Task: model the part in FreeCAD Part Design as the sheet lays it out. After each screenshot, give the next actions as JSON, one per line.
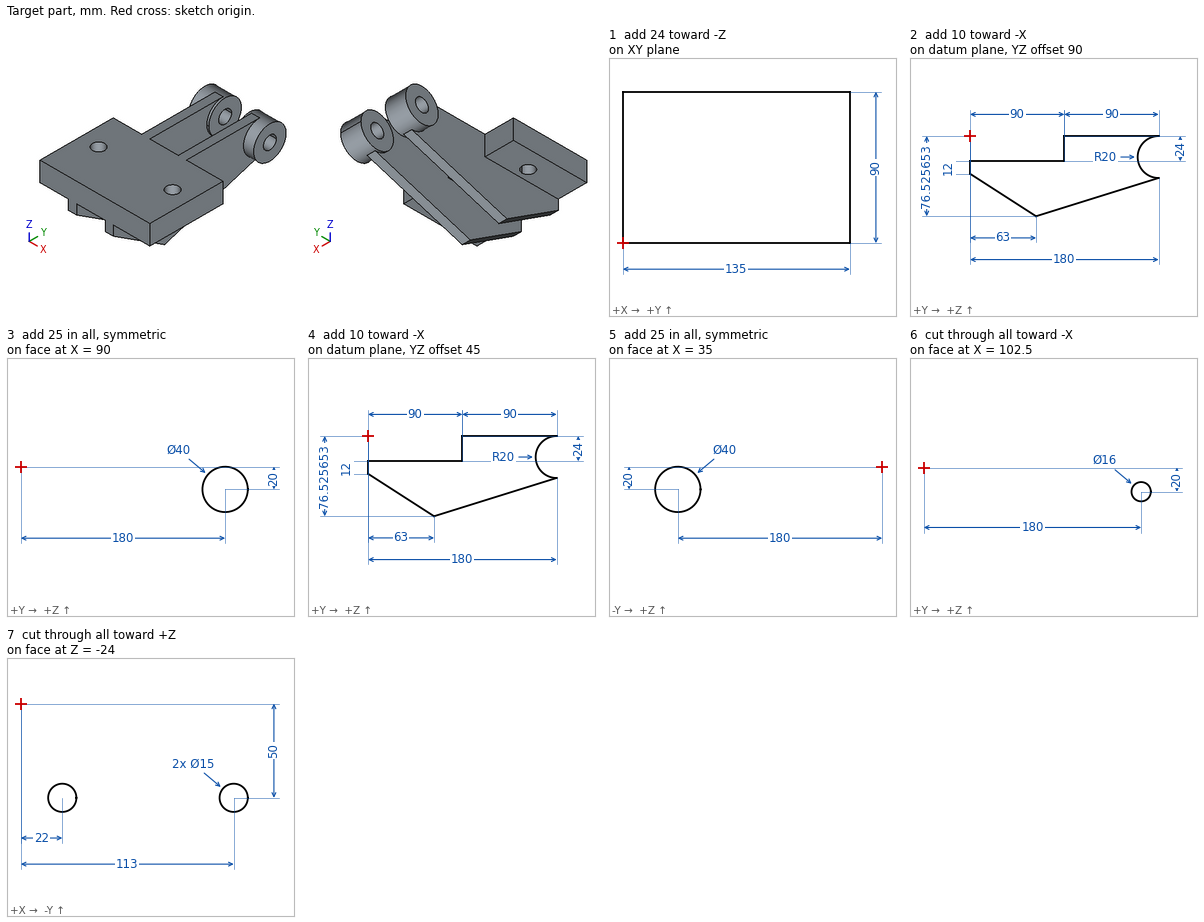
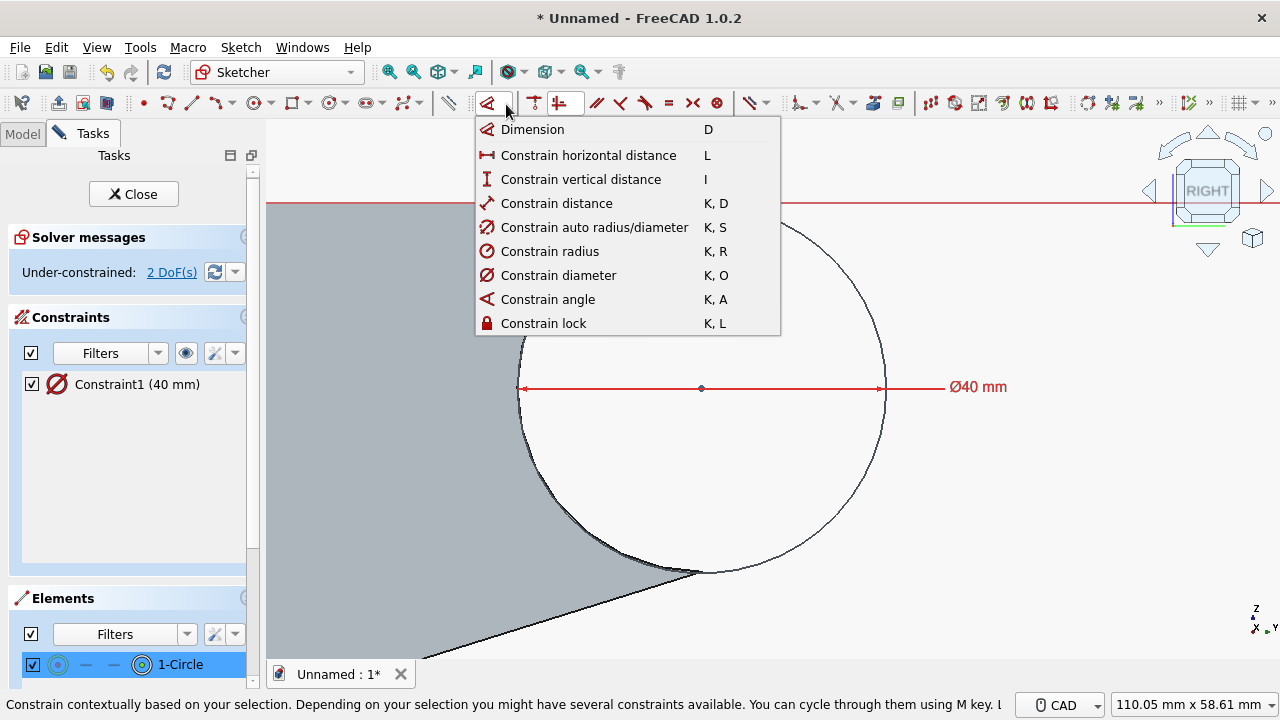
{"action": "left_click", "coordinate": [628, 179]}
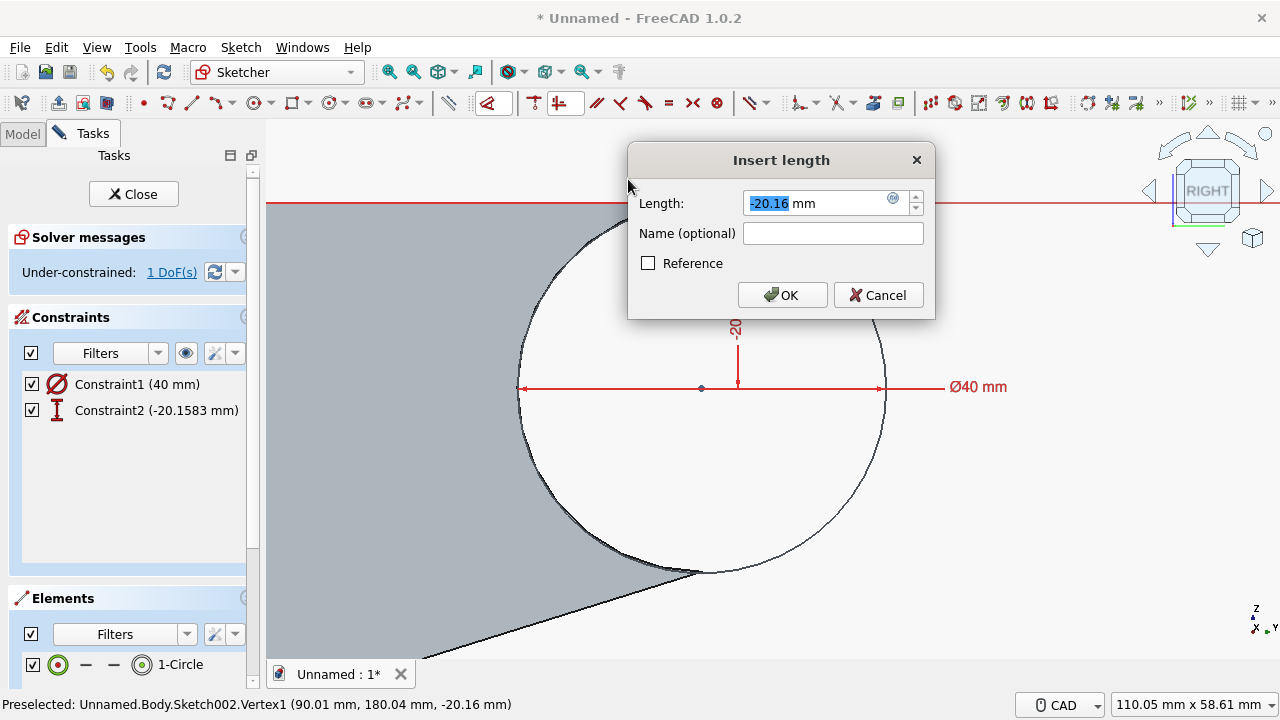
{"action": "type", "text": "-20"}
{"action": "key", "text": "Return"}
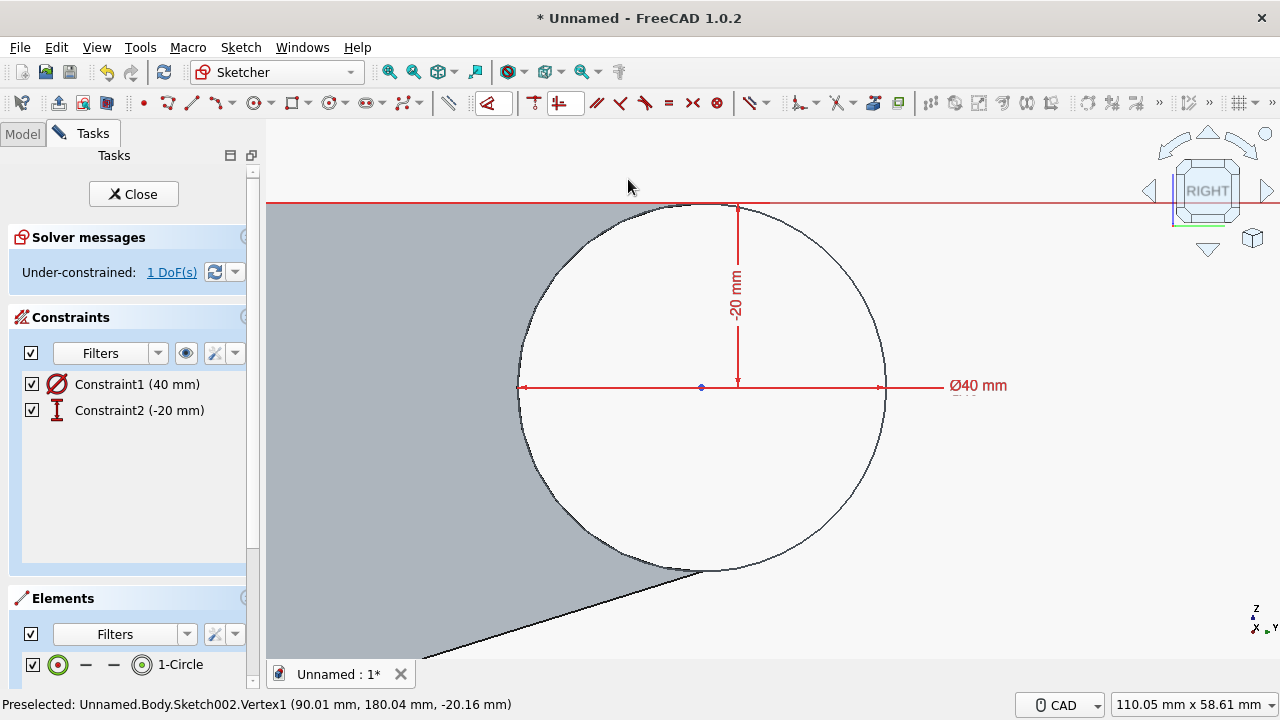
{"action": "left_click", "coordinate": [702, 388]}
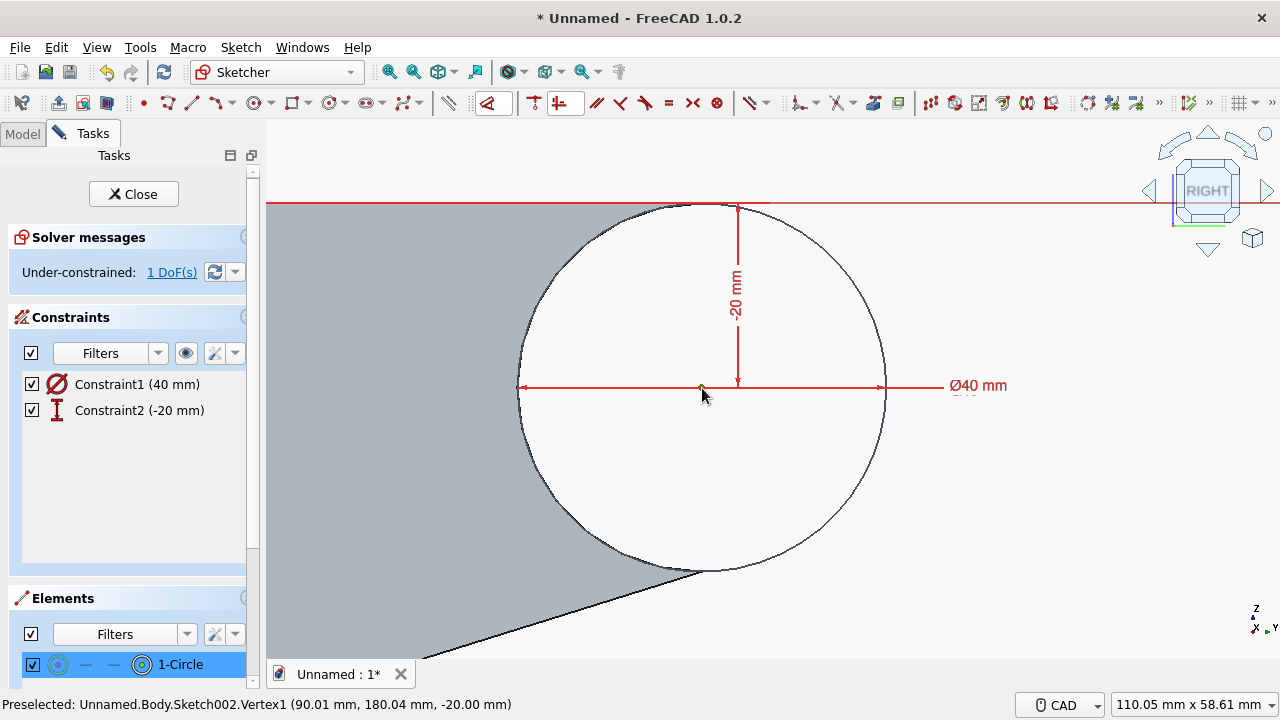
{"action": "key", "text": "l"}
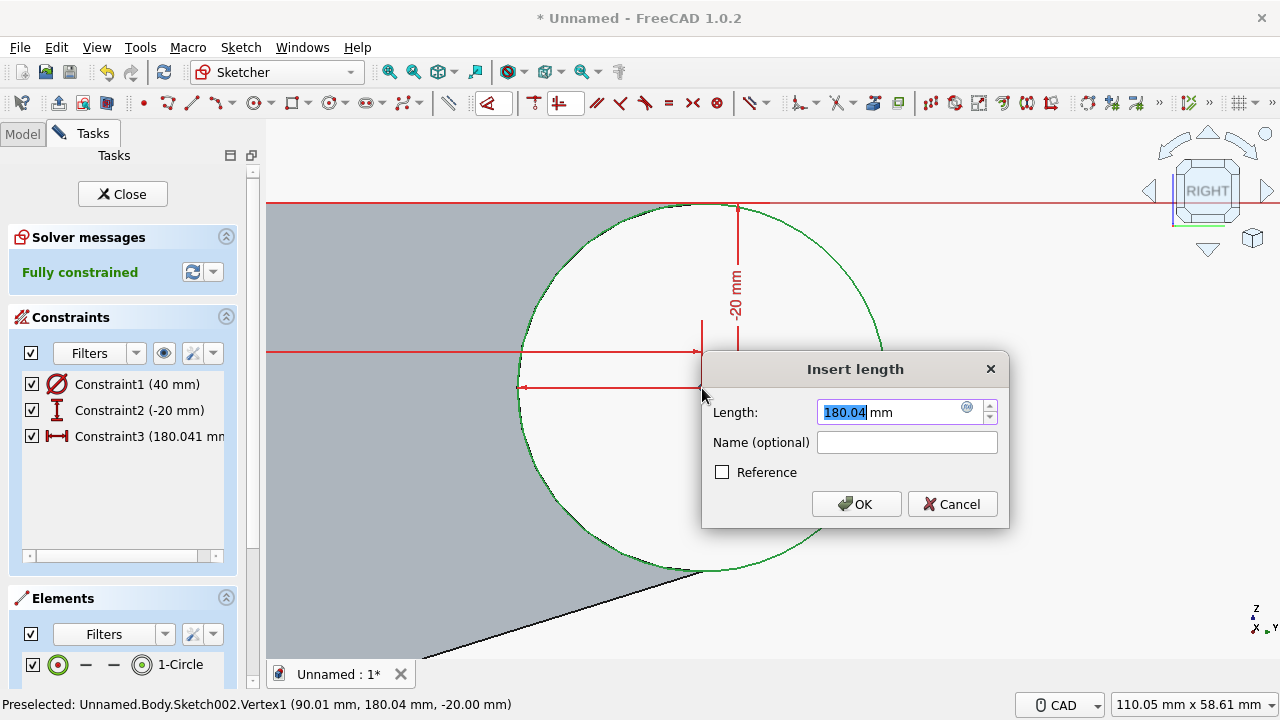
{"action": "type", "text": "180"}
{"action": "key", "text": "Return"}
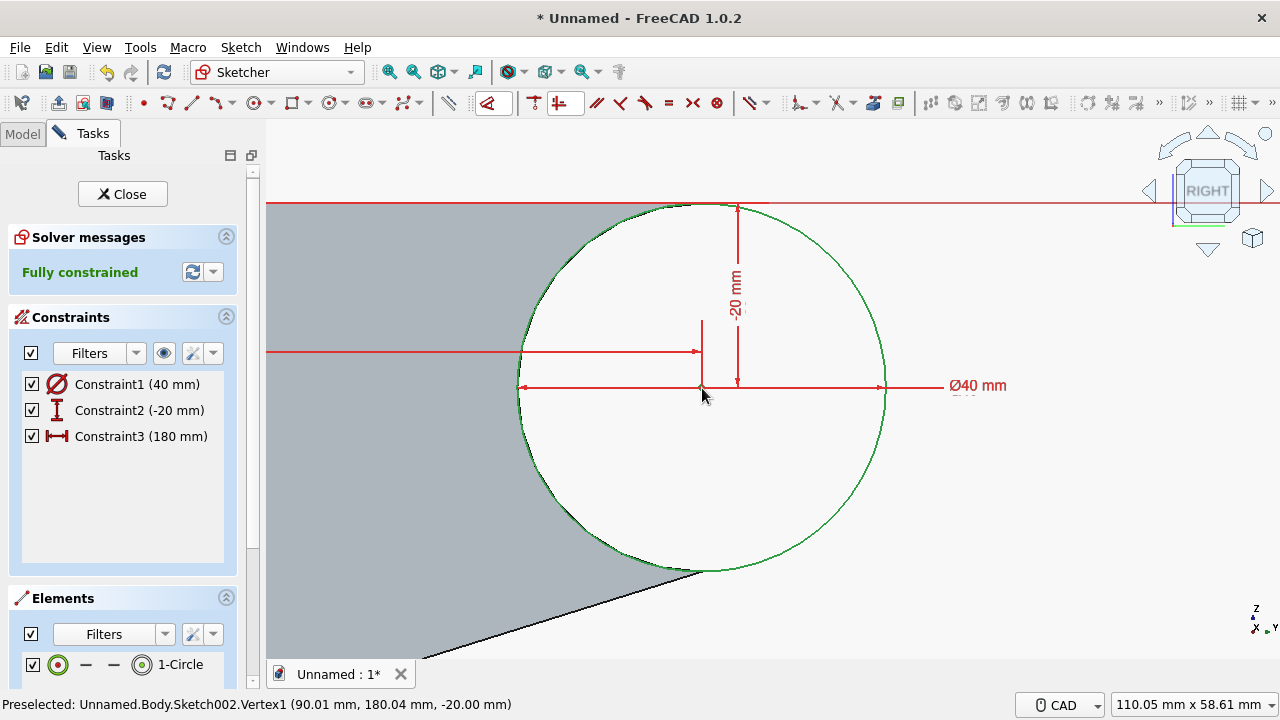
{"action": "left_click", "coordinate": [123, 194]}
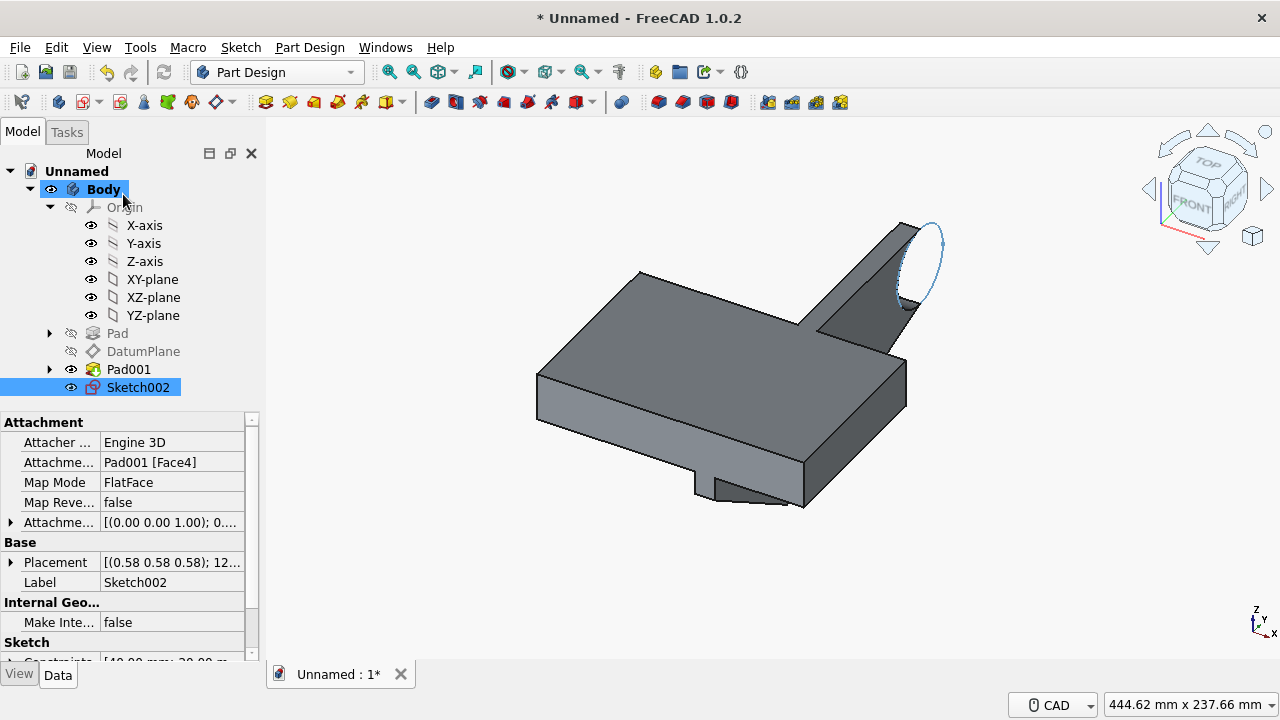
{"action": "left_click", "coordinate": [266, 102]}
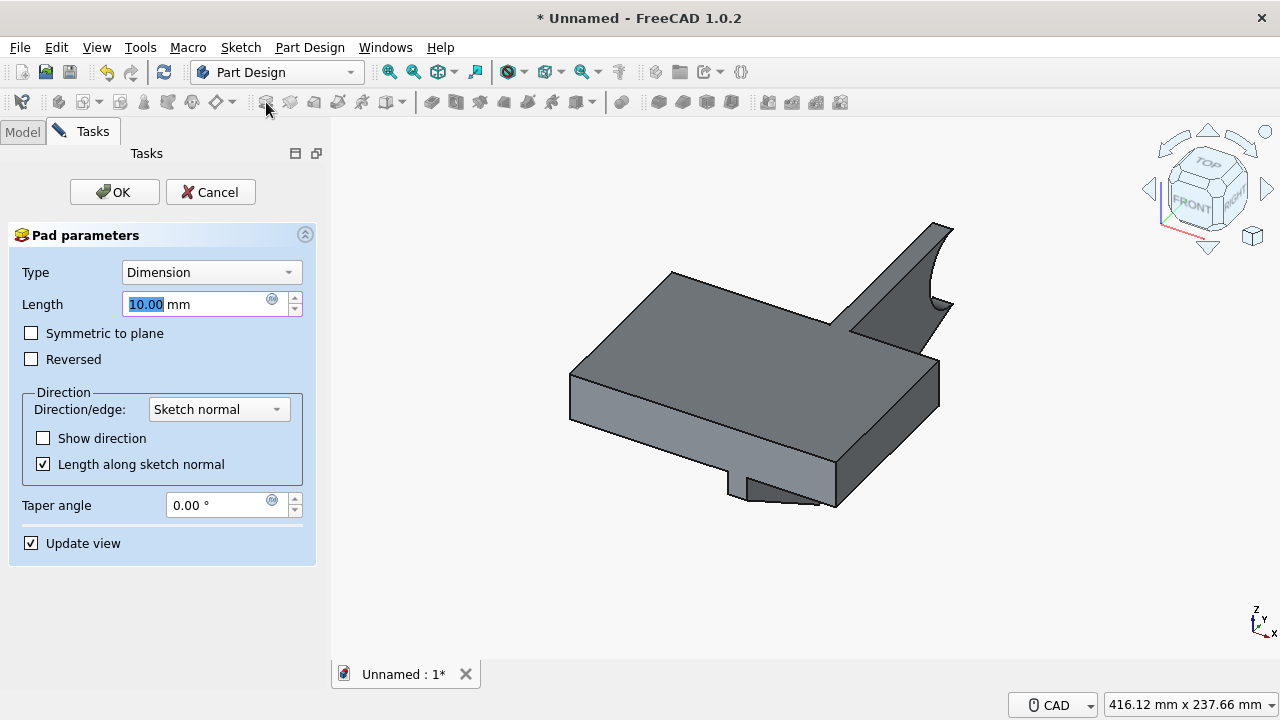
{"action": "type", "text": "25"}
{"action": "key", "text": "Tab"}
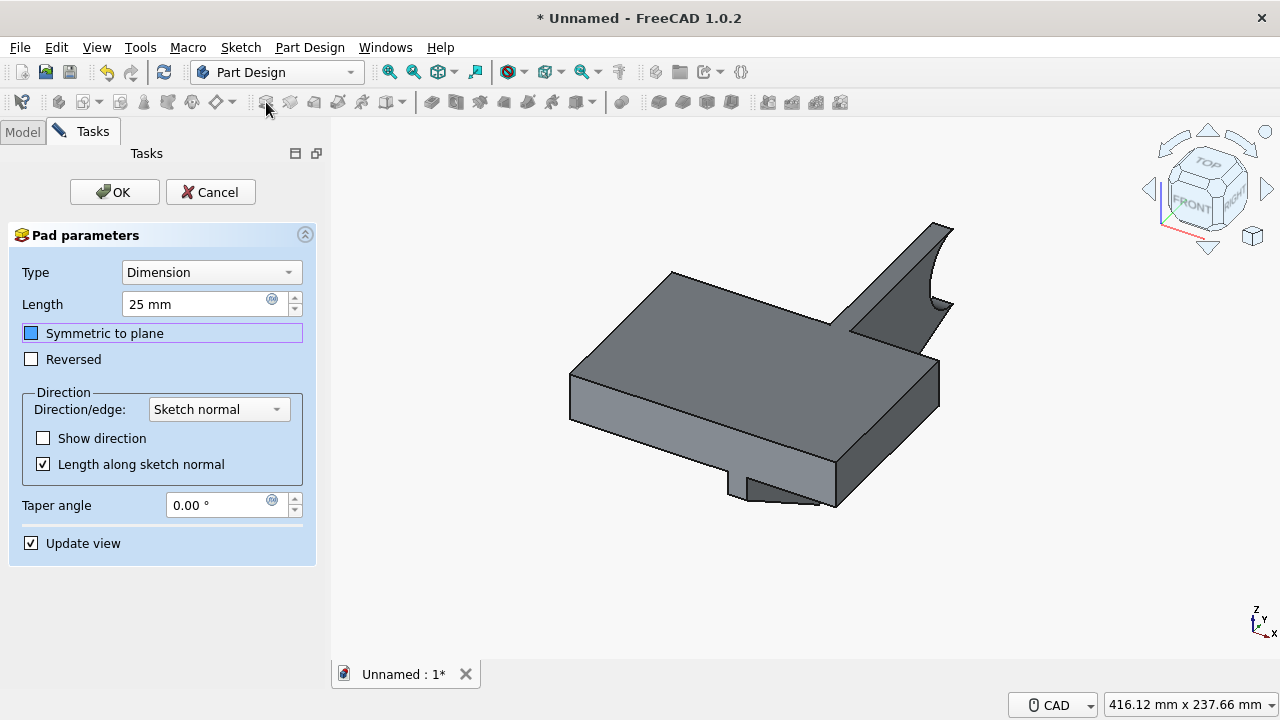
{"action": "left_click", "coordinate": [30, 333]}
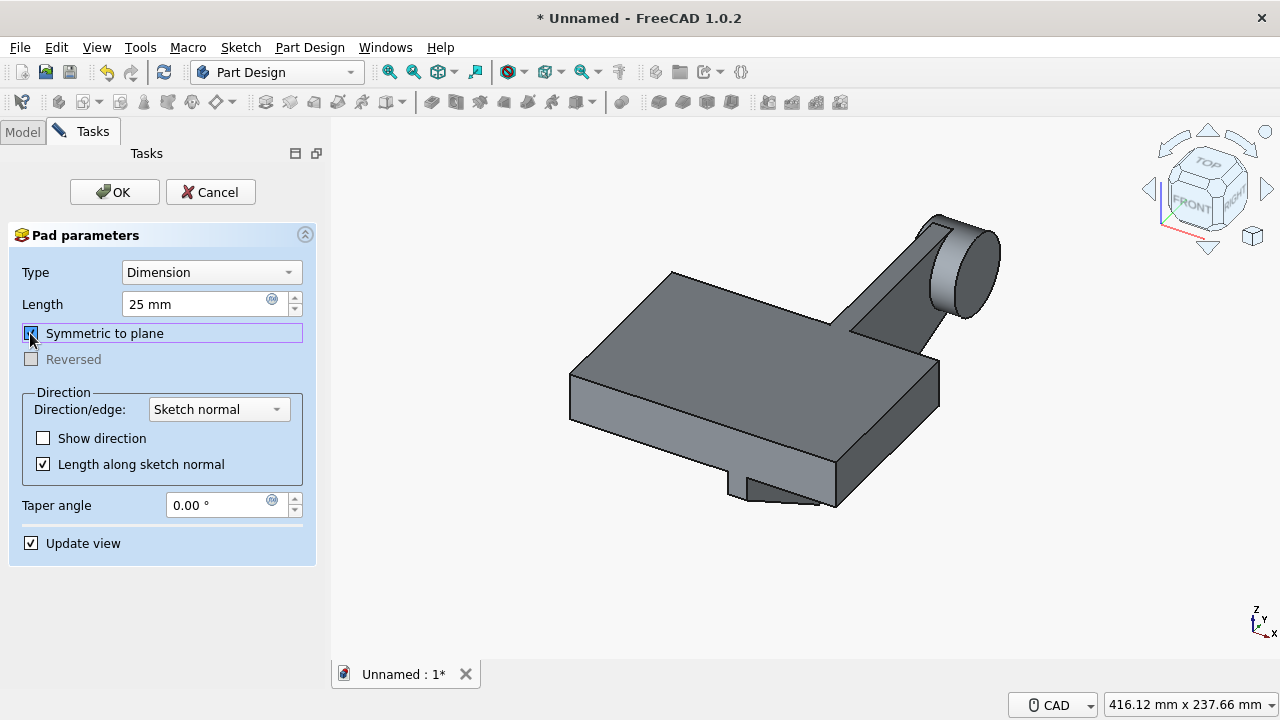
{"action": "left_click", "coordinate": [115, 192]}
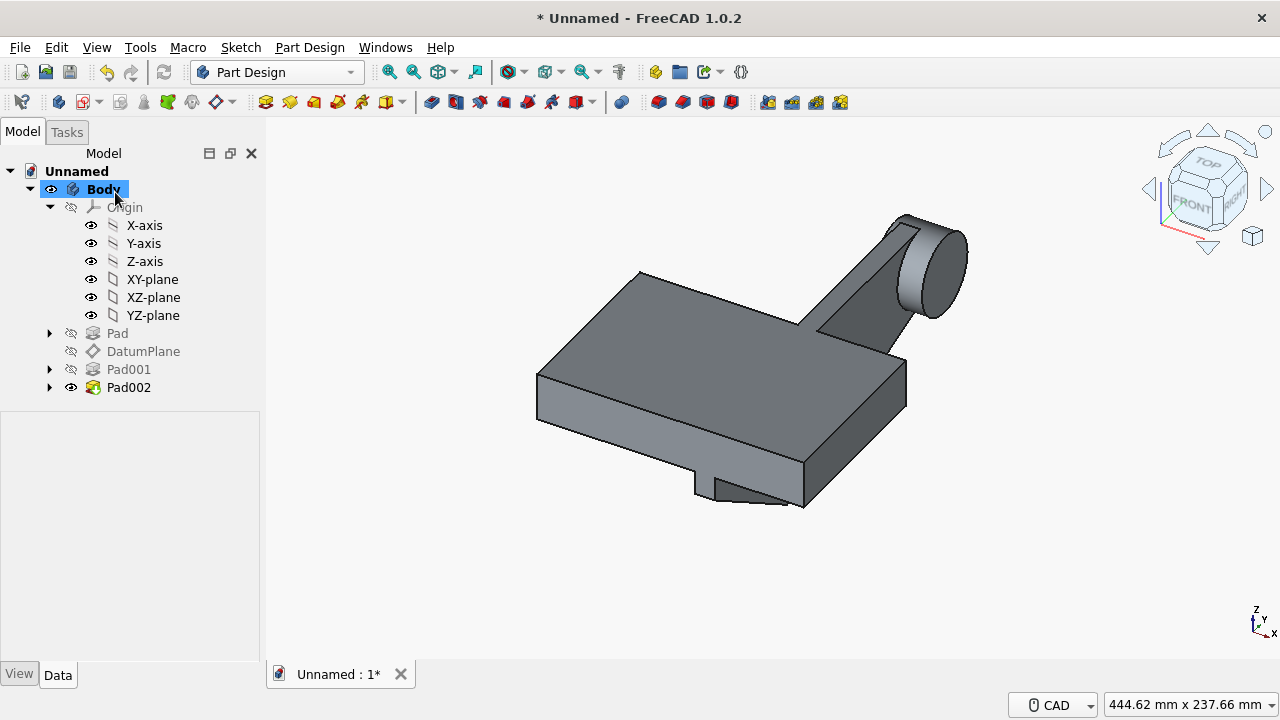
{"action": "left_click", "coordinate": [136, 315]}